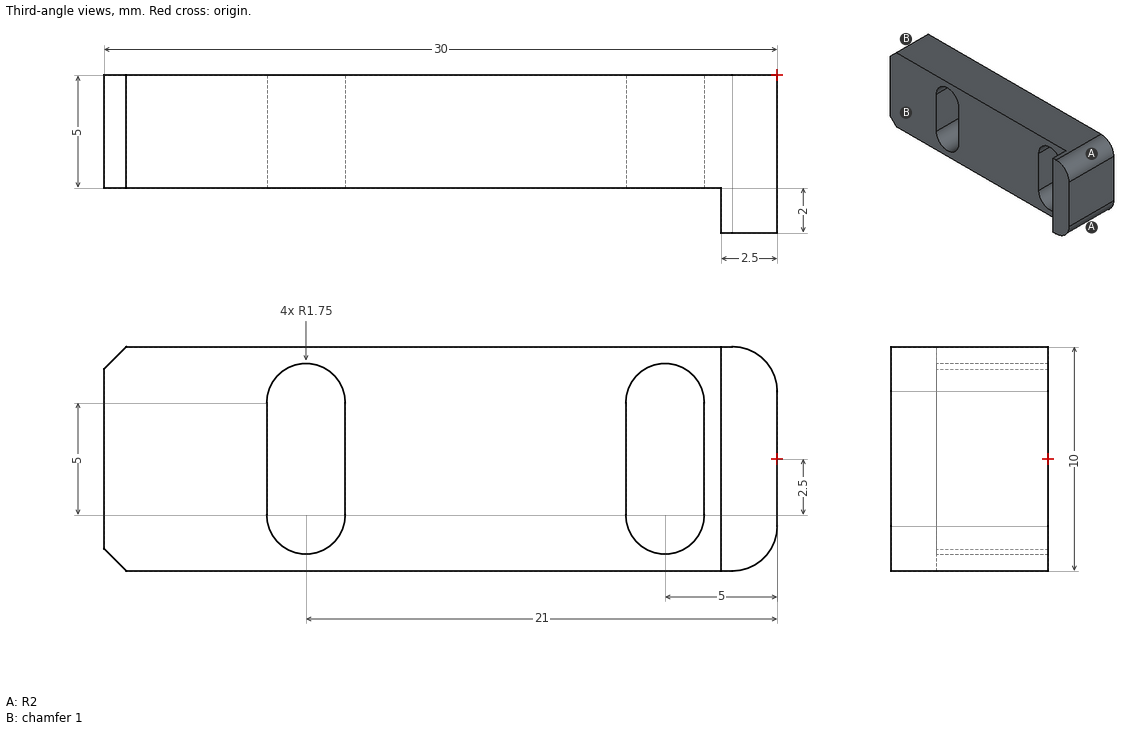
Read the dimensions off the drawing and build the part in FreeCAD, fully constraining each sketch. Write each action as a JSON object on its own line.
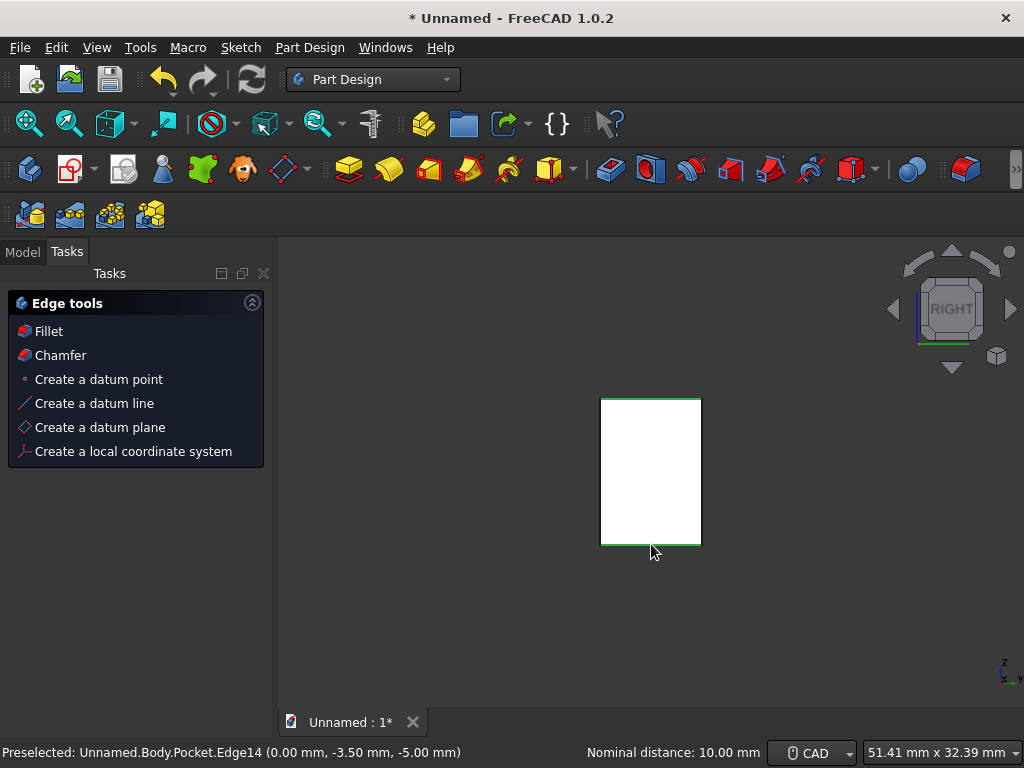
{"action": "left_click", "coordinate": [966, 170]}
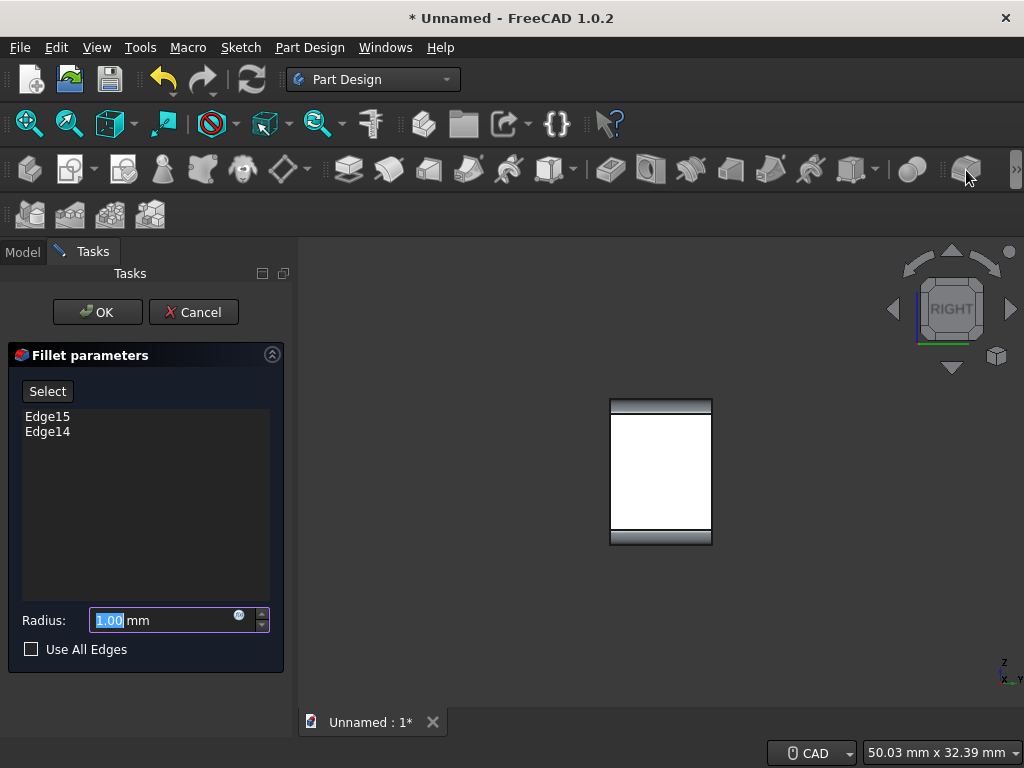
{"action": "type", "text": "2"}
{"action": "key", "text": "Tab"}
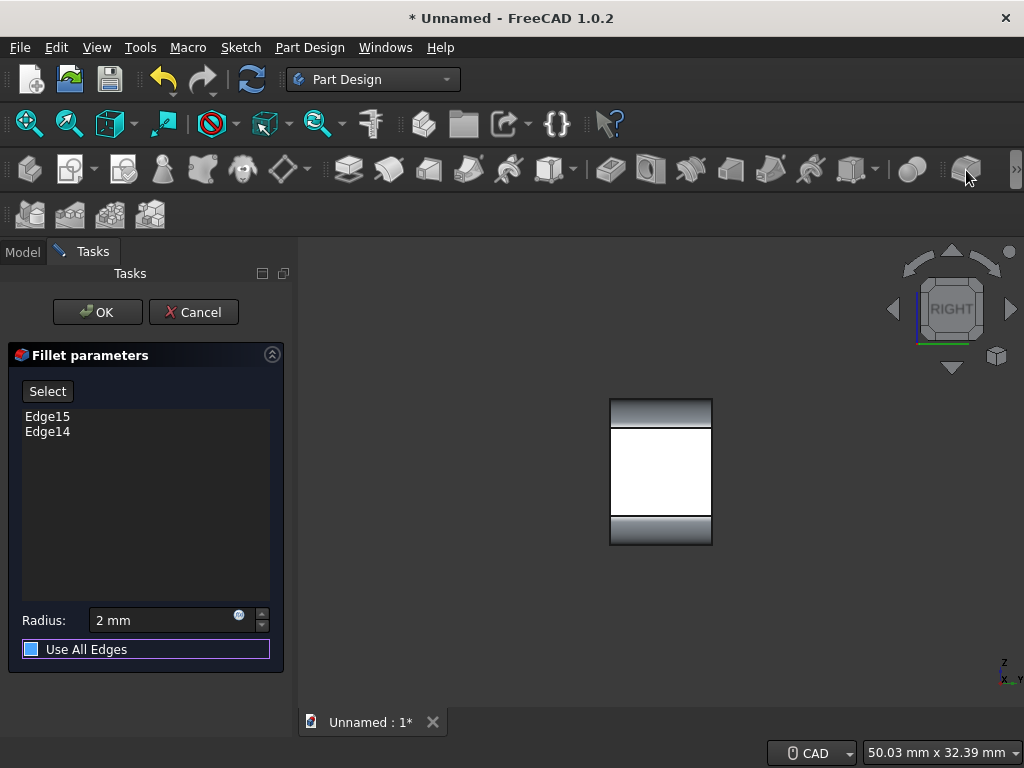
{"action": "left_click", "coordinate": [98, 312]}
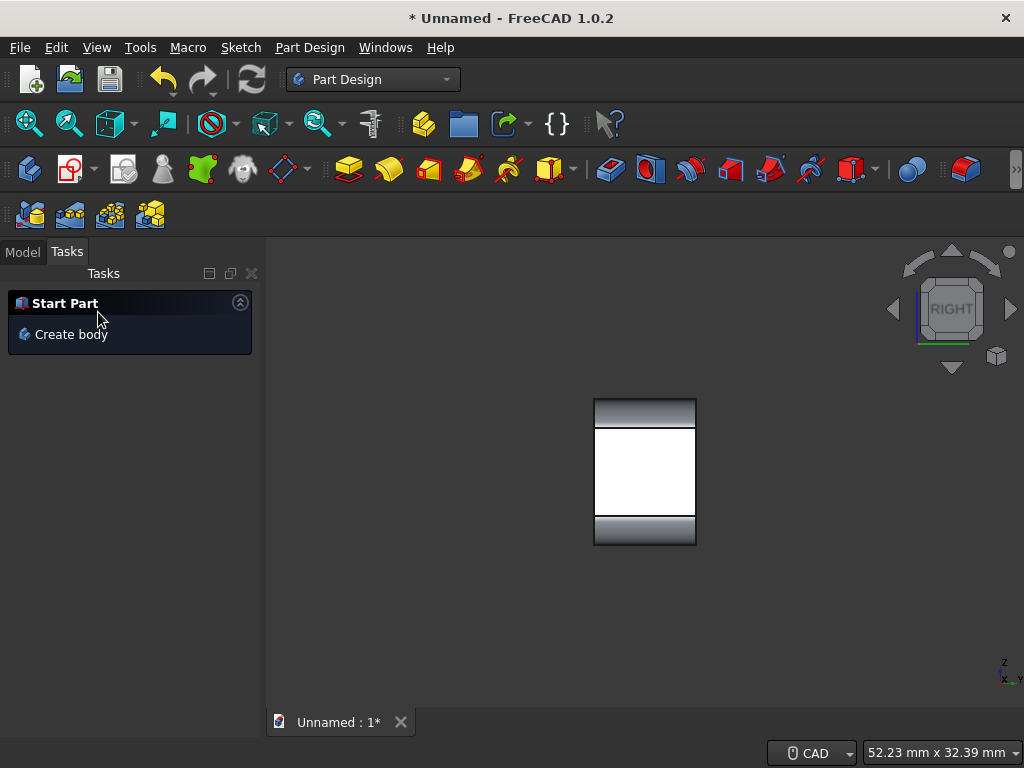
{"action": "left_click", "coordinate": [30, 124]}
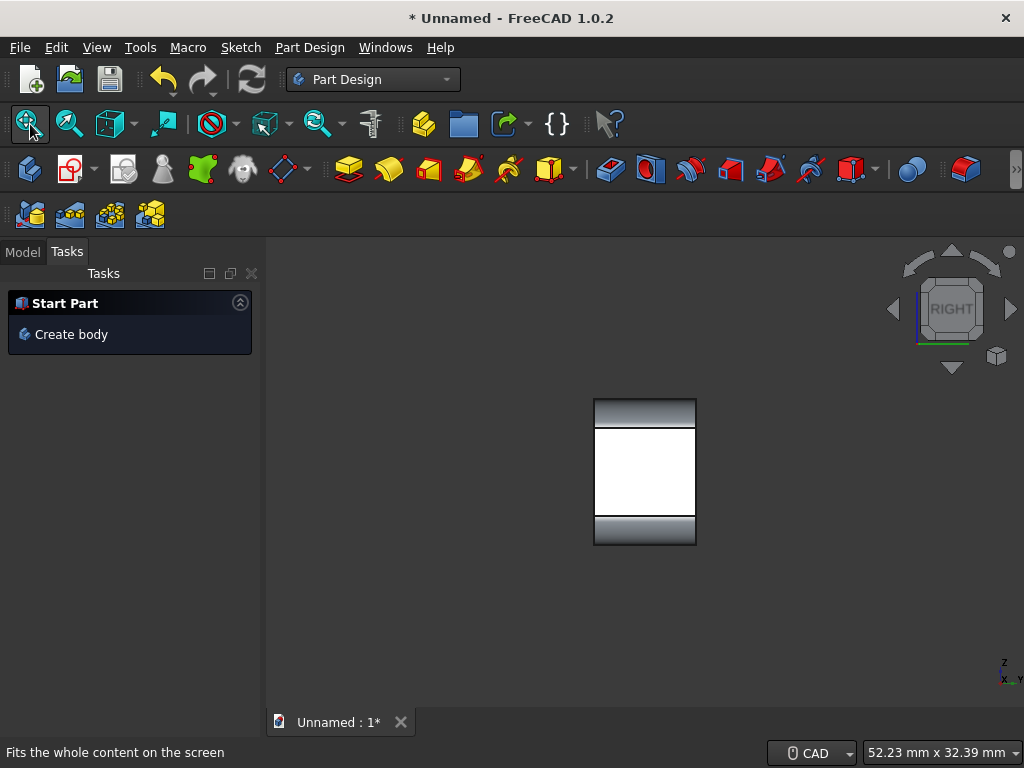
{"action": "key", "text": "0"}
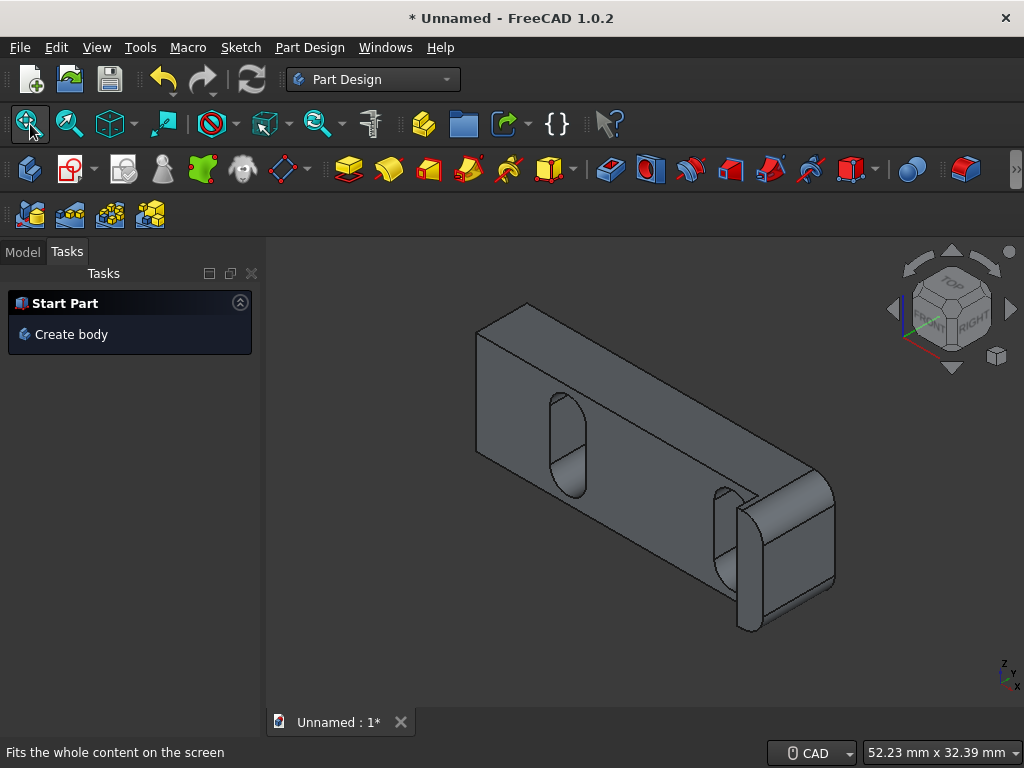
{"action": "key", "text": "2"}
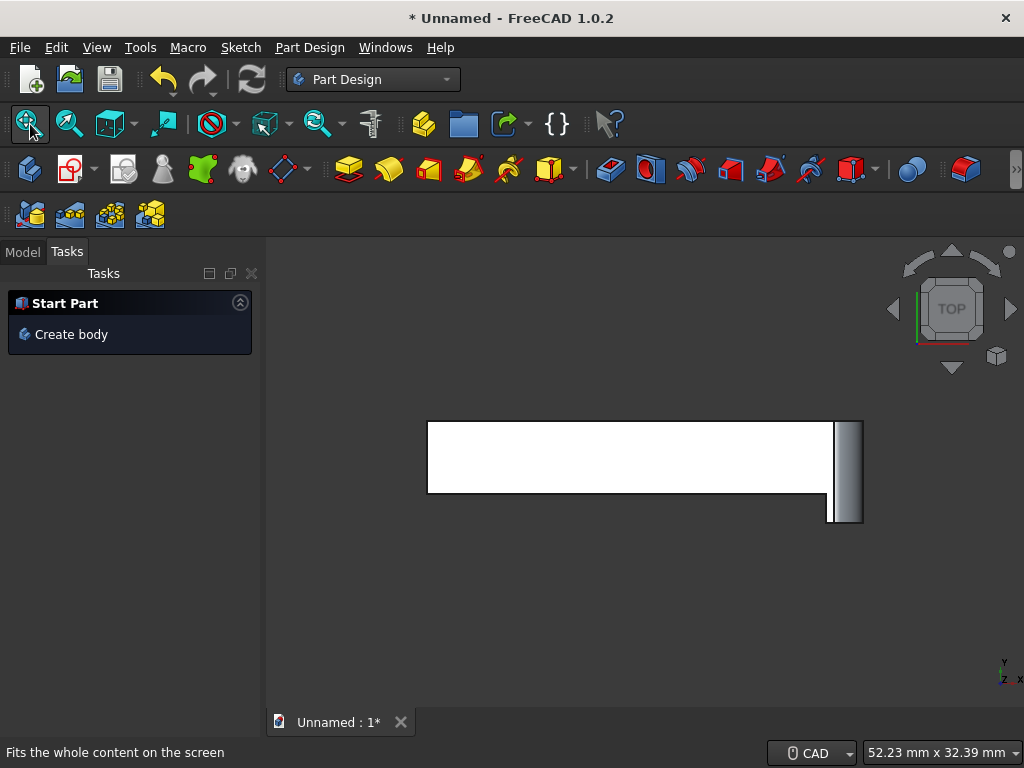
{"action": "left_click", "coordinate": [427, 456]}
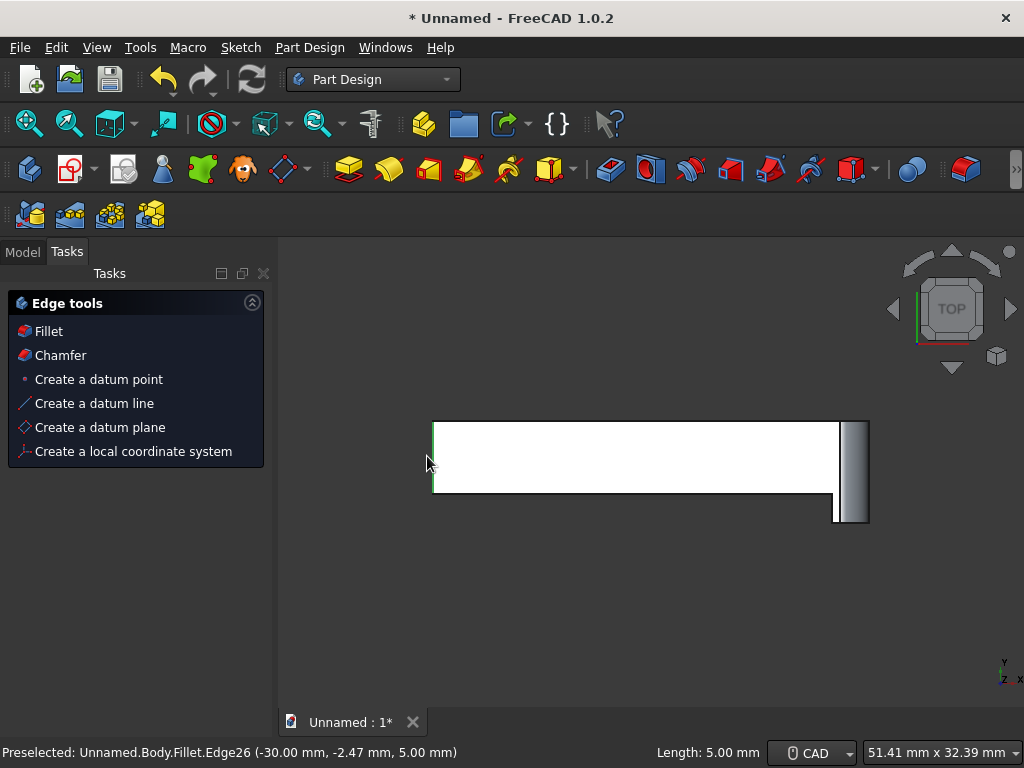
{"action": "key", "text": "1"}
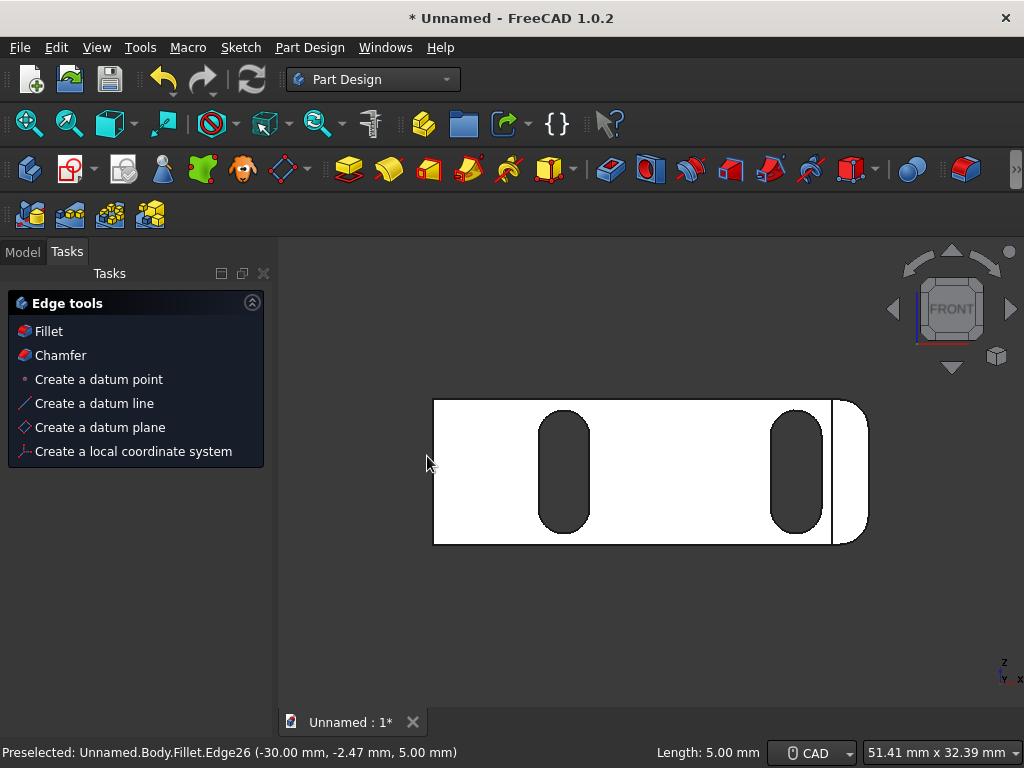
{"action": "key", "text": "3"}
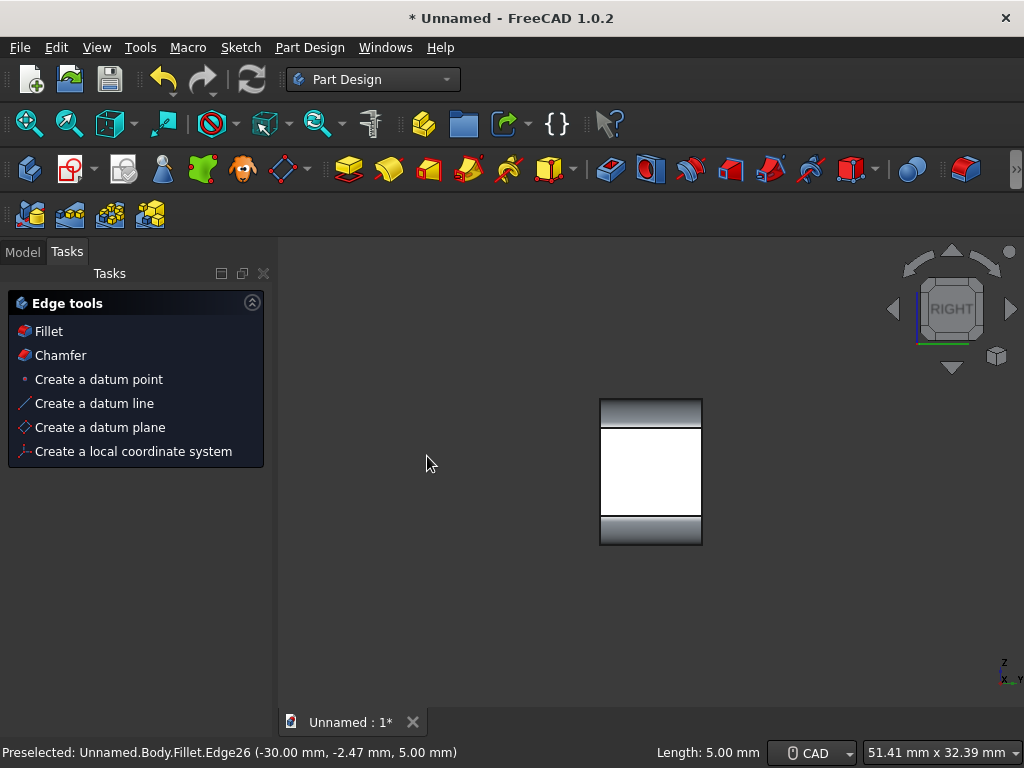
{"action": "left_click", "coordinate": [30, 124]}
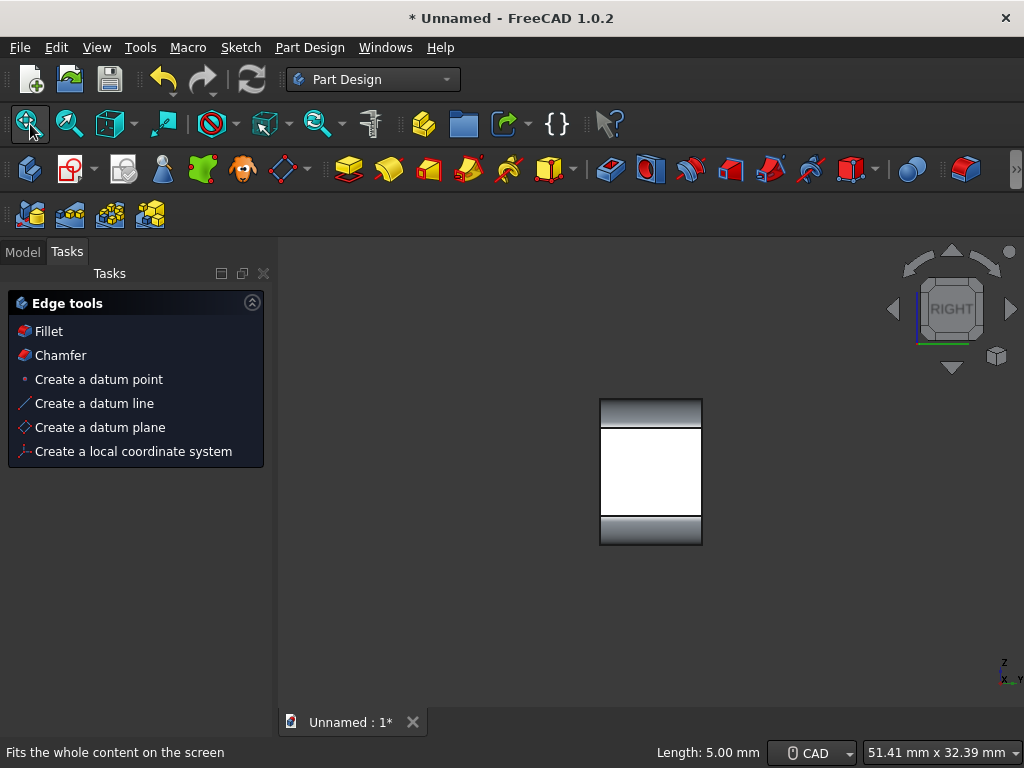
{"action": "key", "text": "5"}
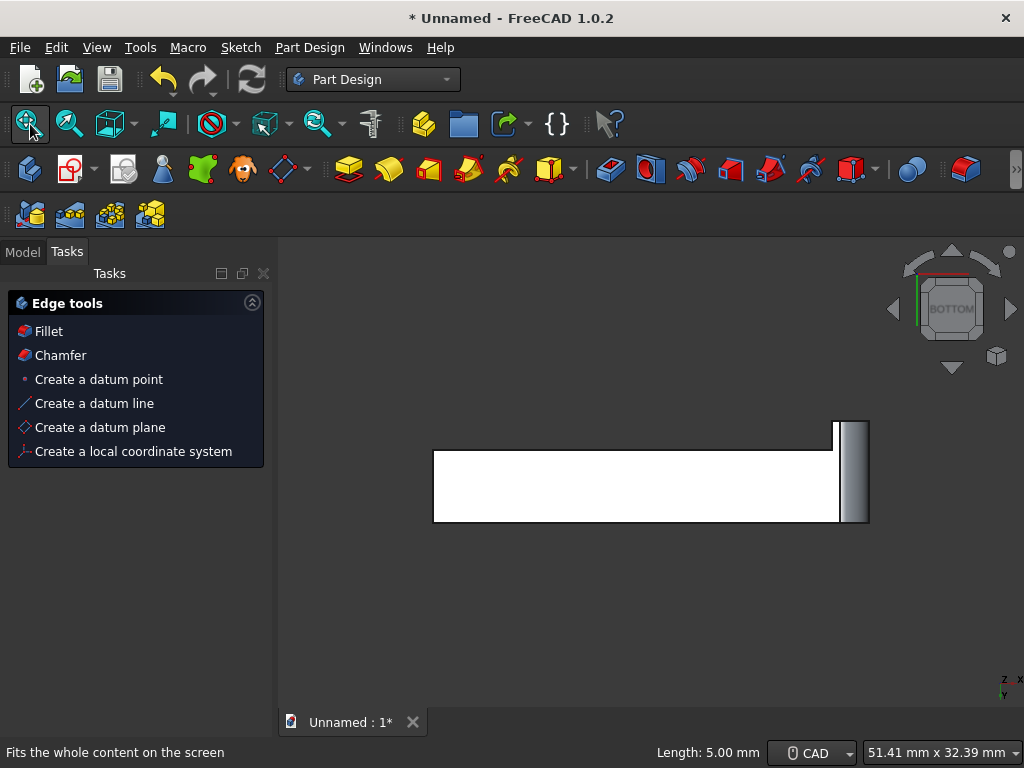
{"action": "left_click", "coordinate": [433, 486], "text": "ctrl"}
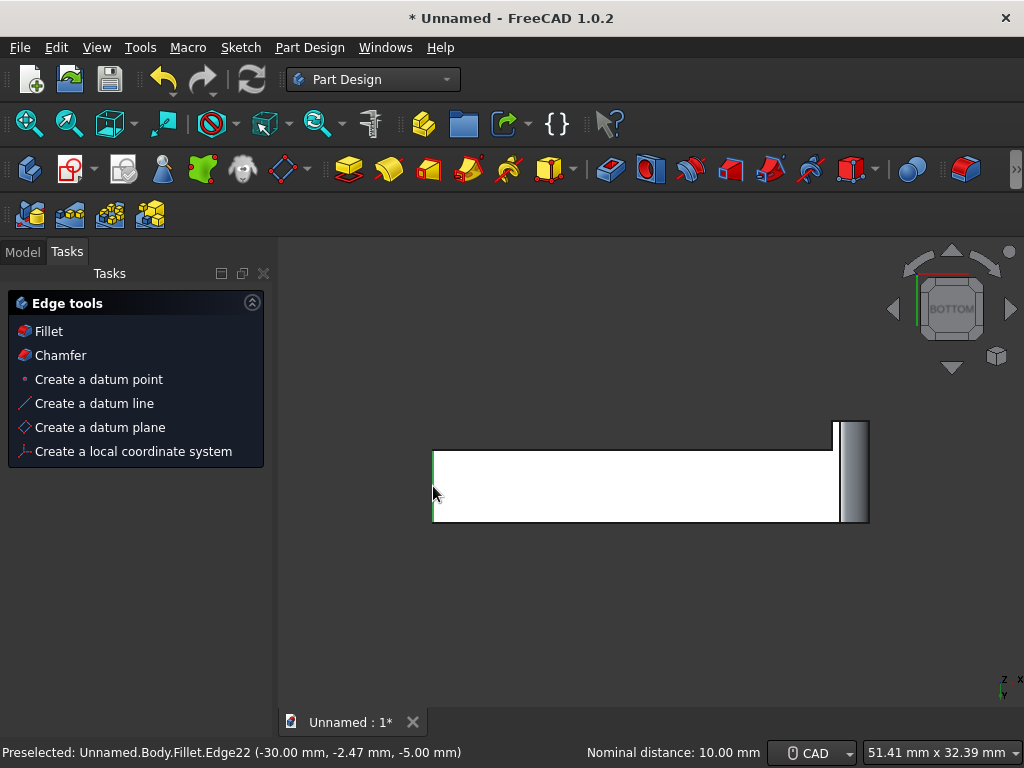
{"action": "left_click", "coordinate": [136, 355]}